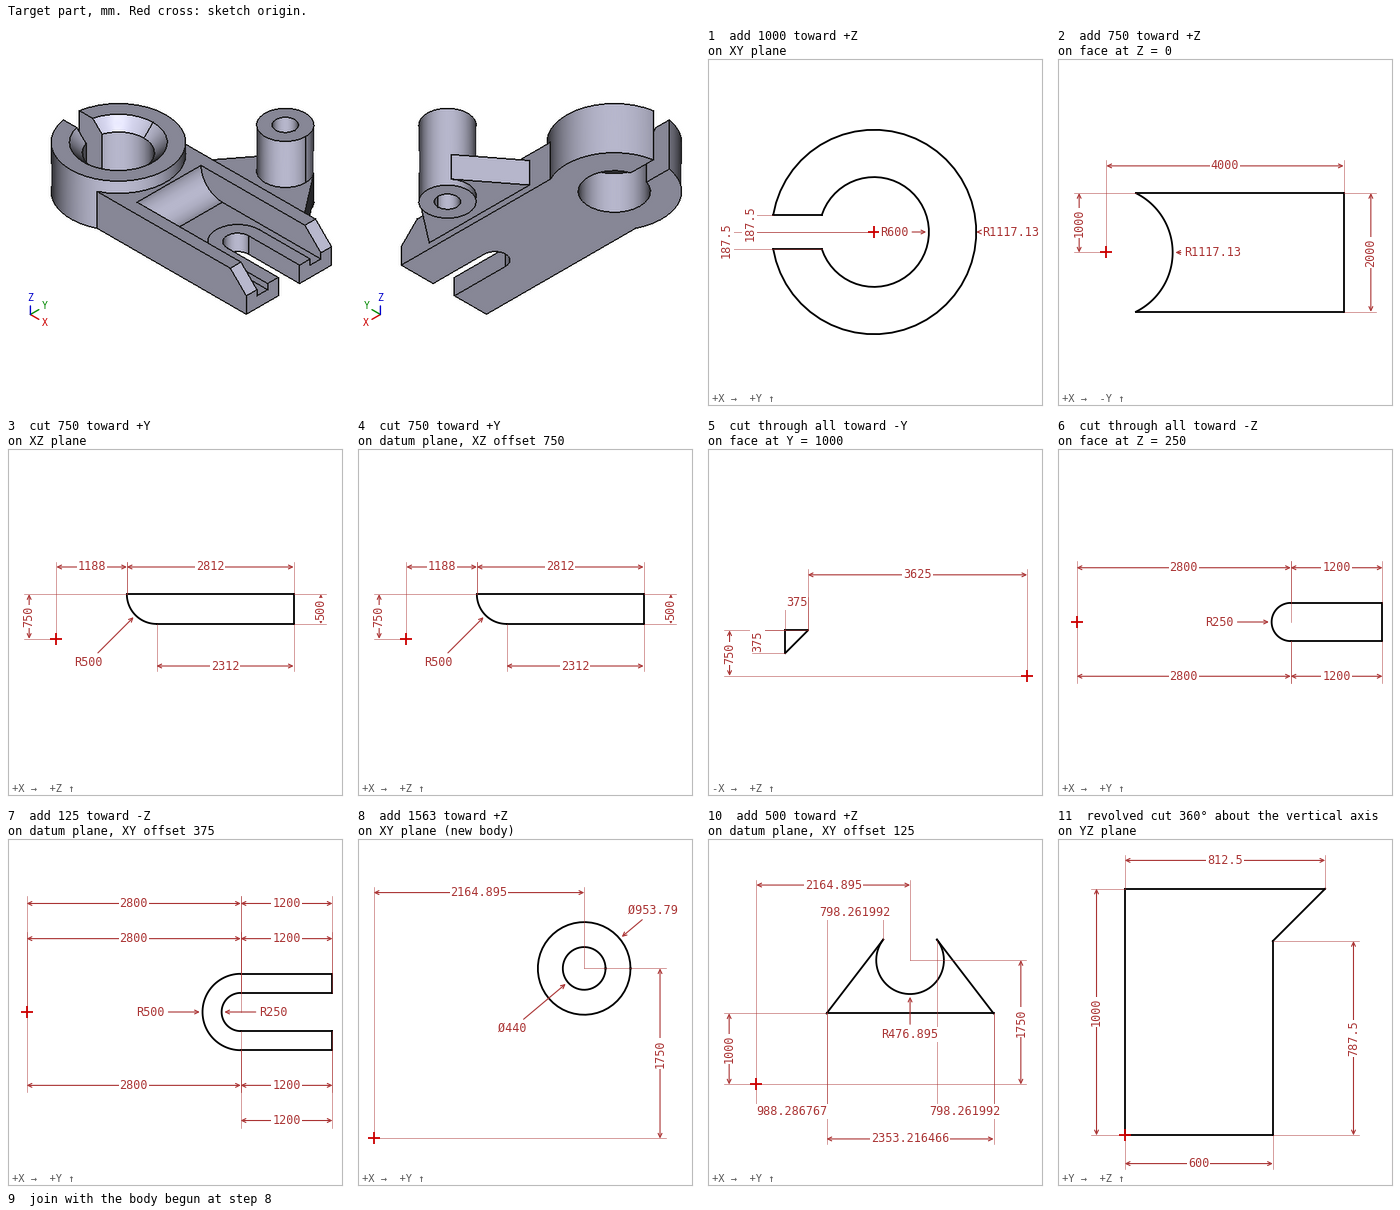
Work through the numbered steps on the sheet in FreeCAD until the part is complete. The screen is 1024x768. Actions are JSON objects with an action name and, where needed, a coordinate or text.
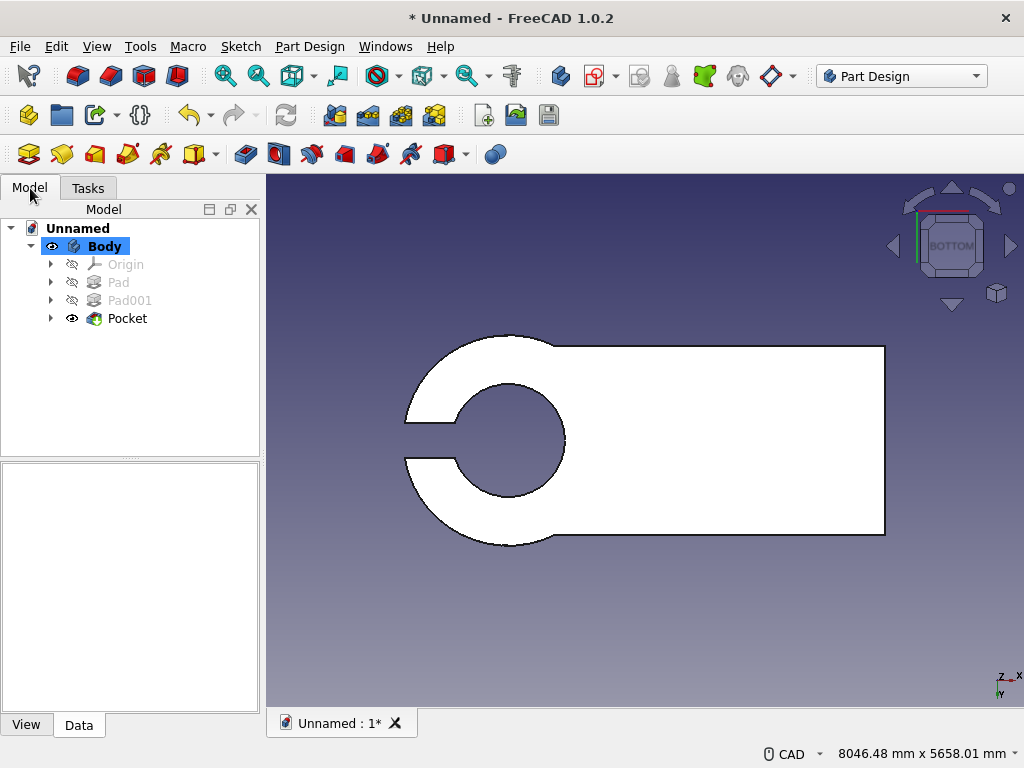
{"action": "left_click", "coordinate": [51, 264]}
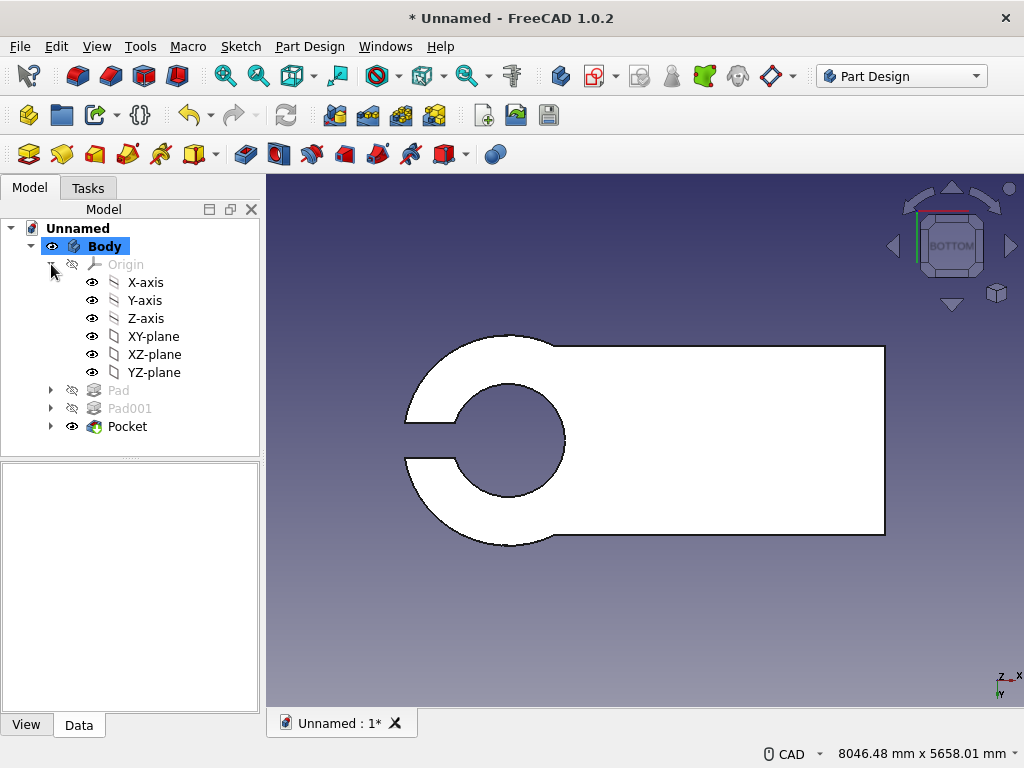
{"action": "left_click", "coordinate": [137, 354]}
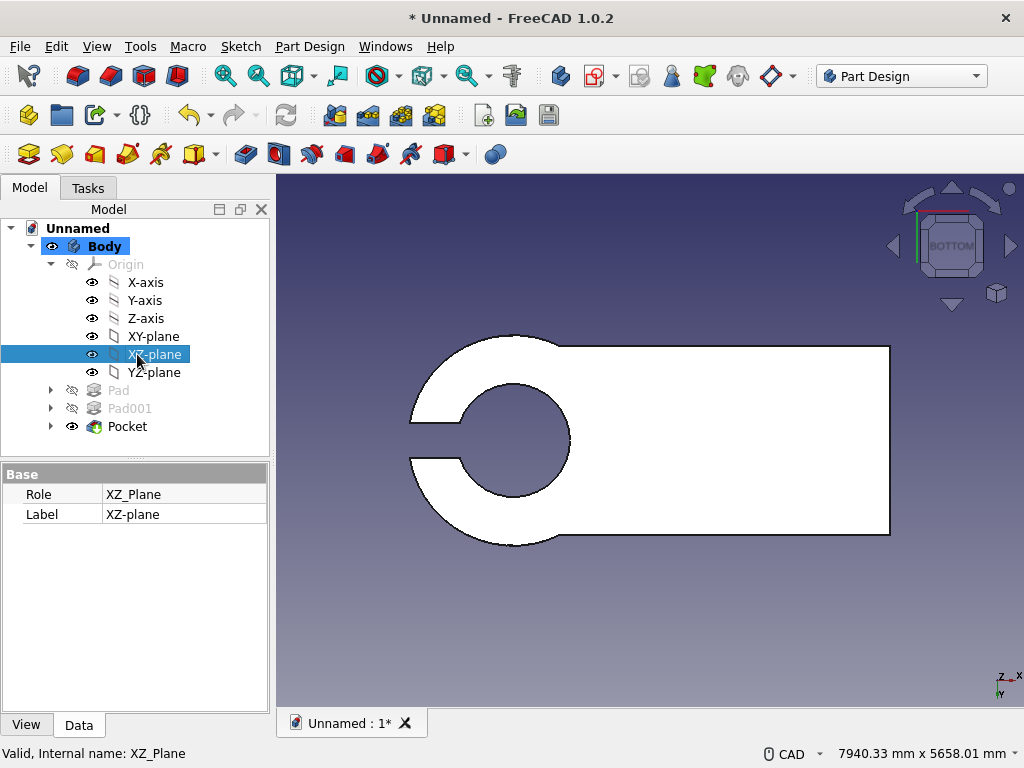
{"action": "left_click", "coordinate": [770, 76]}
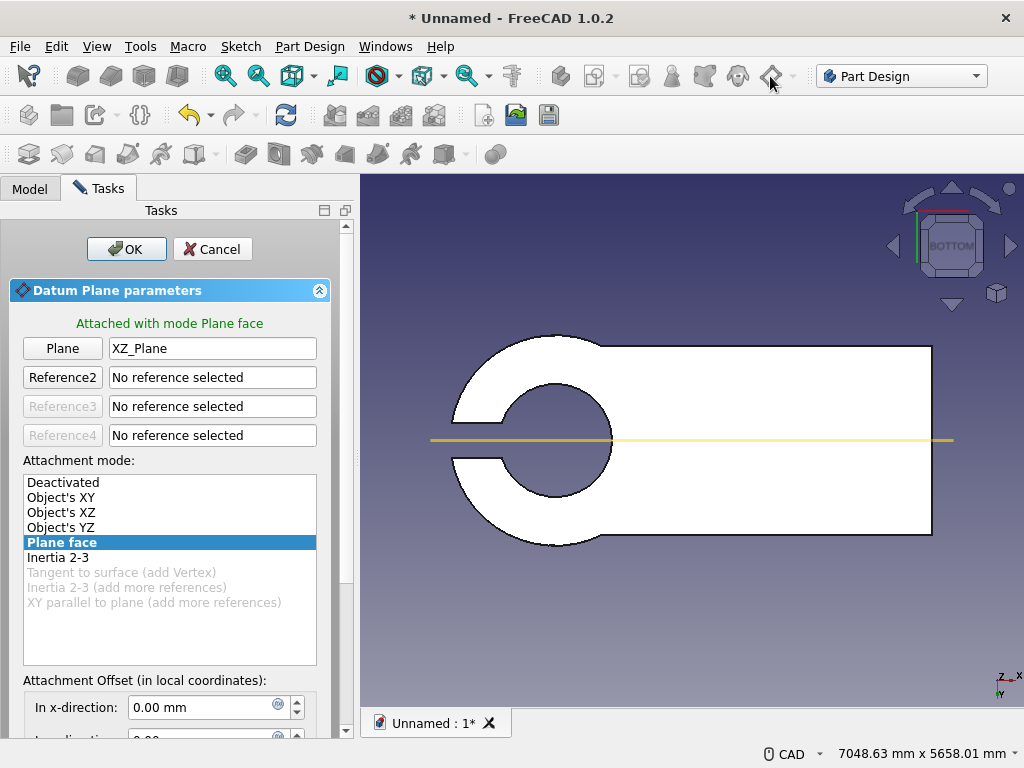
{"action": "scroll", "coordinate": [346, 479], "scroll_direction": "down", "scroll_amount": 2}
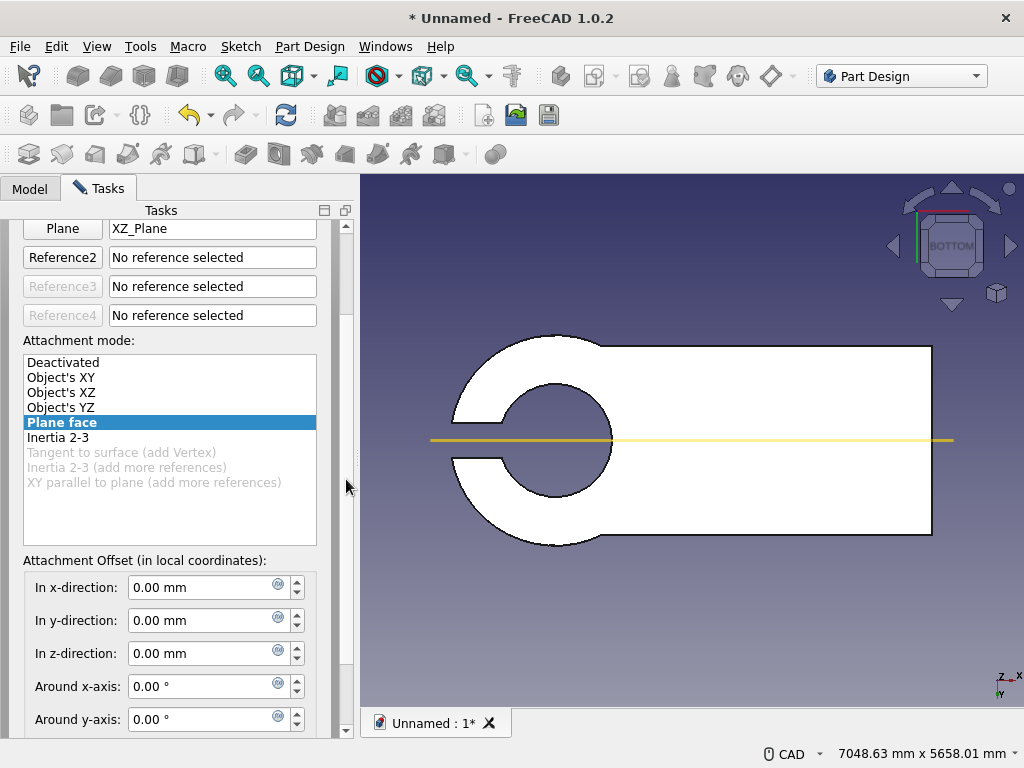
{"action": "triple_click", "coordinate": [210, 654]}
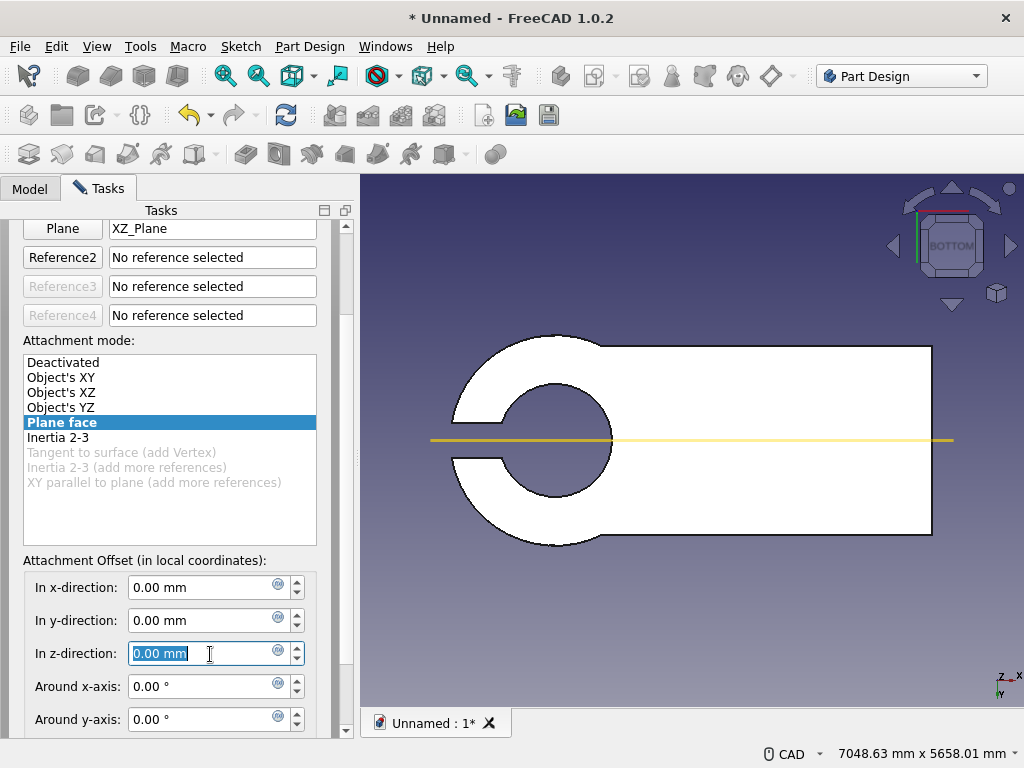
{"action": "type", "text": "750"}
{"action": "key", "text": "Tab"}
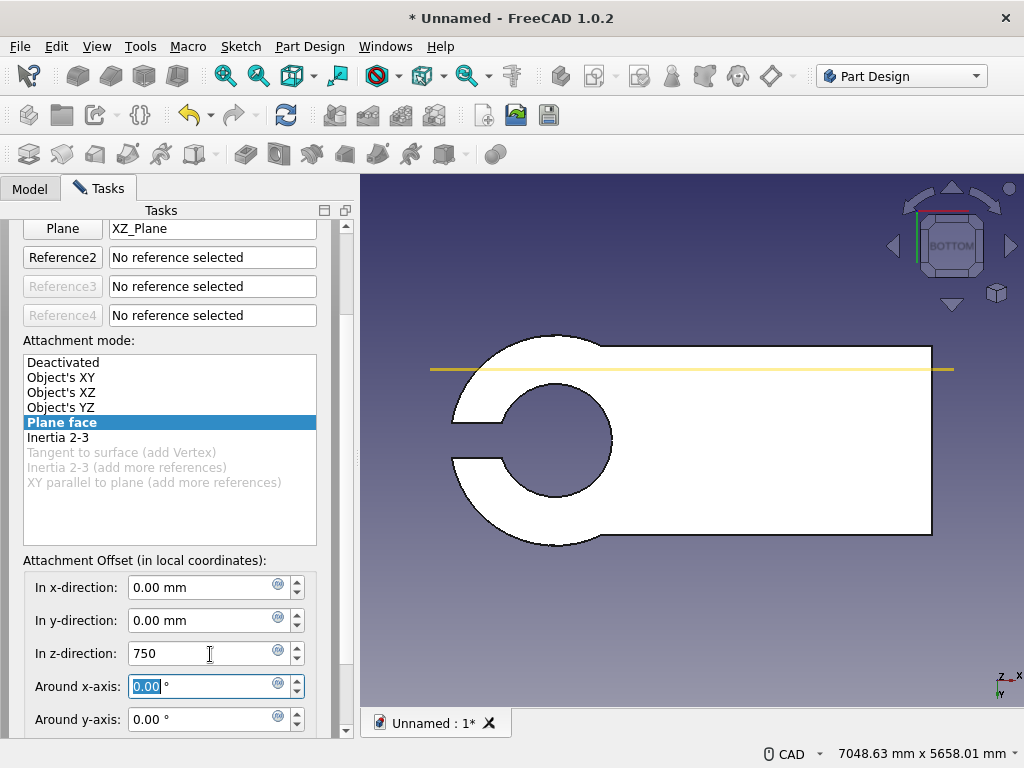
{"action": "scroll", "coordinate": [346, 479], "scroll_direction": "up", "scroll_amount": 3}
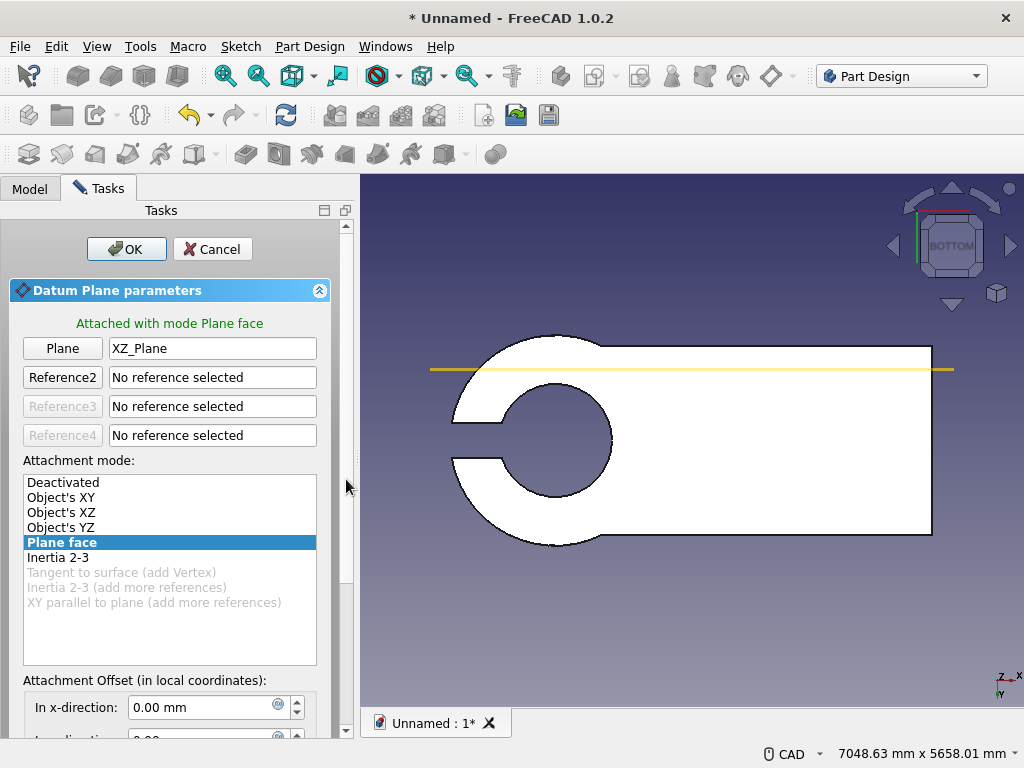
{"action": "left_click", "coordinate": [127, 249]}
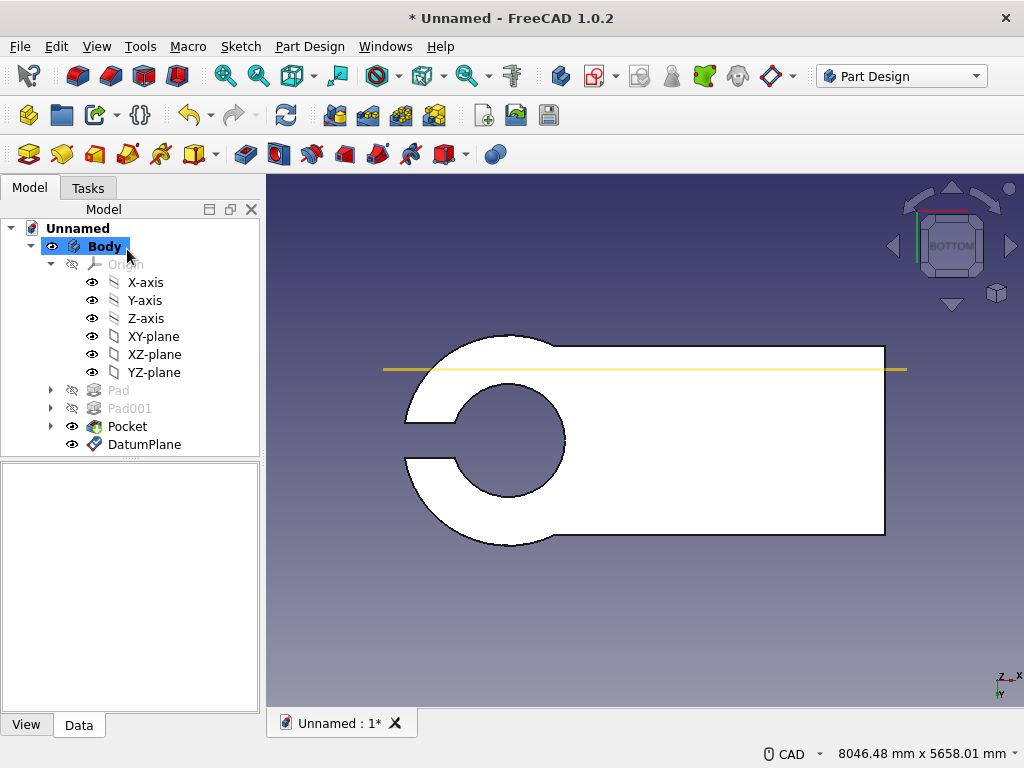
{"action": "left_click", "coordinate": [117, 444]}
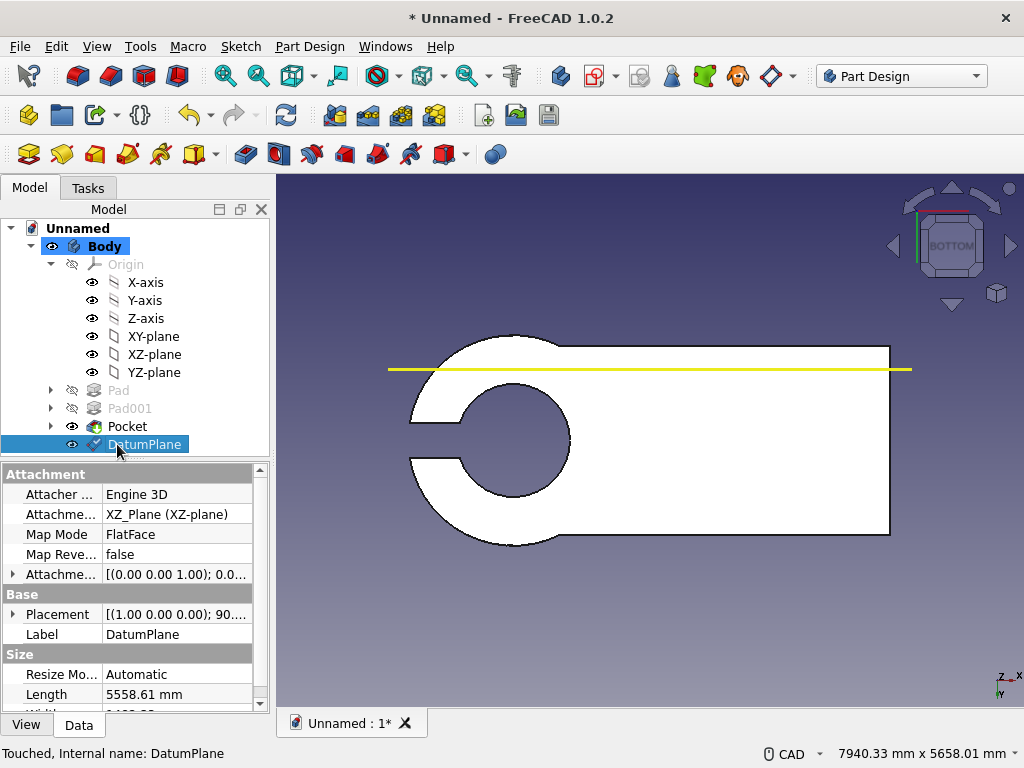
{"action": "left_click", "coordinate": [594, 76]}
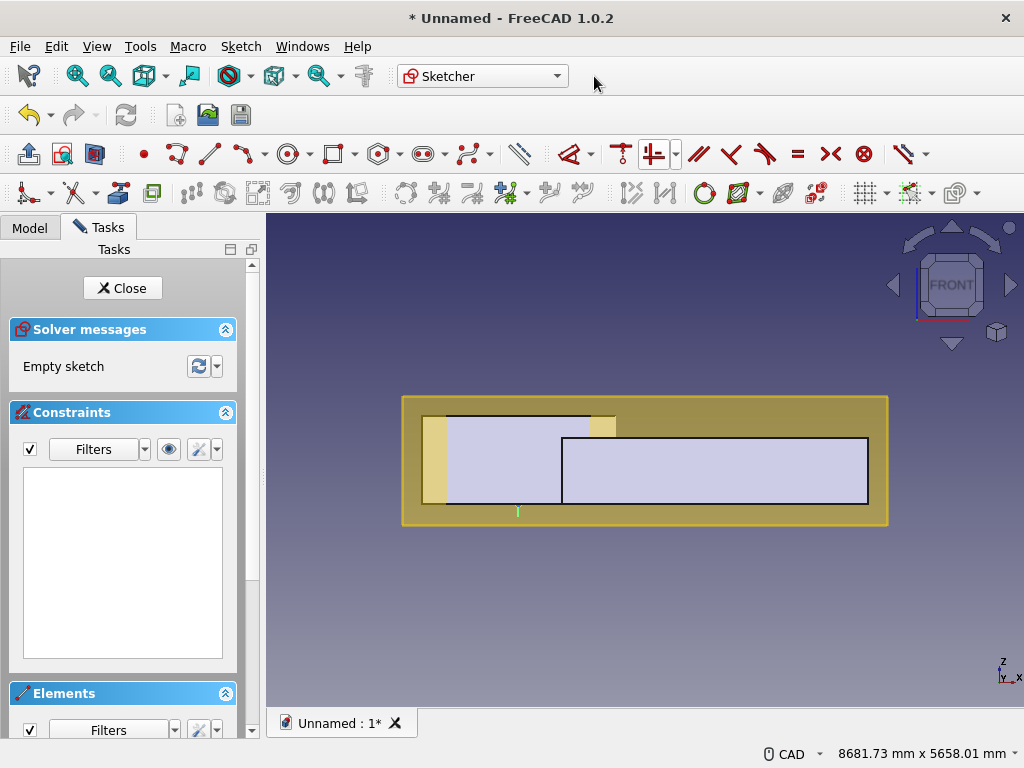
{"action": "key", "text": "q s"}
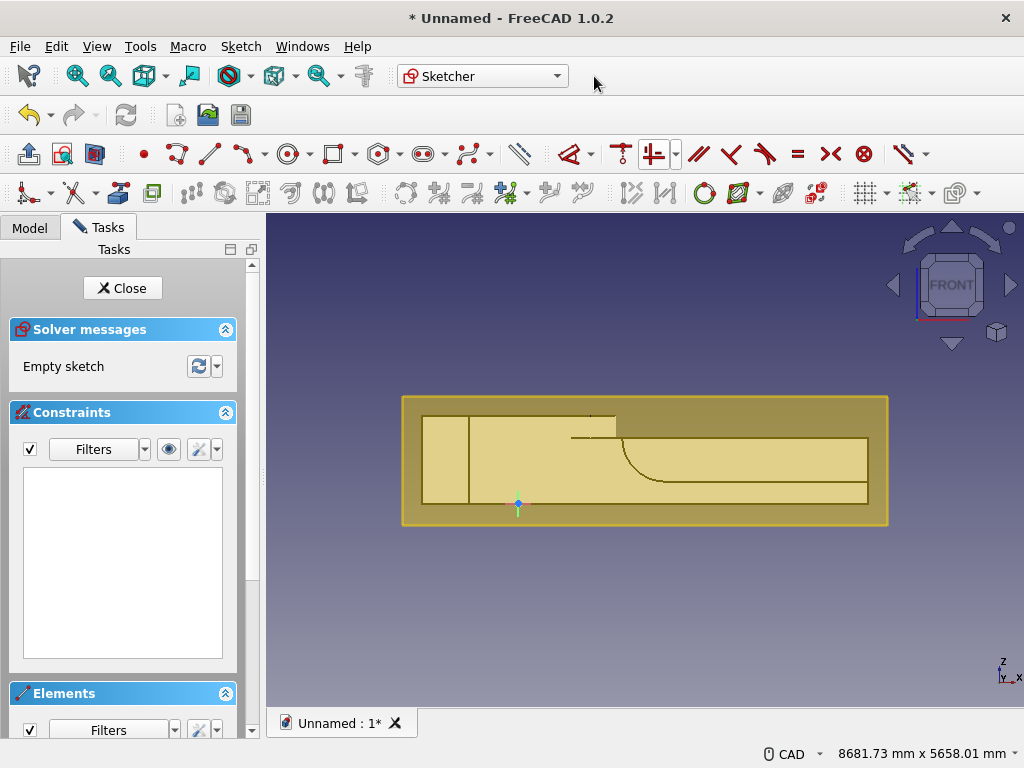
{"action": "scroll", "coordinate": [294, 411], "scroll_direction": "down", "scroll_amount": 1}